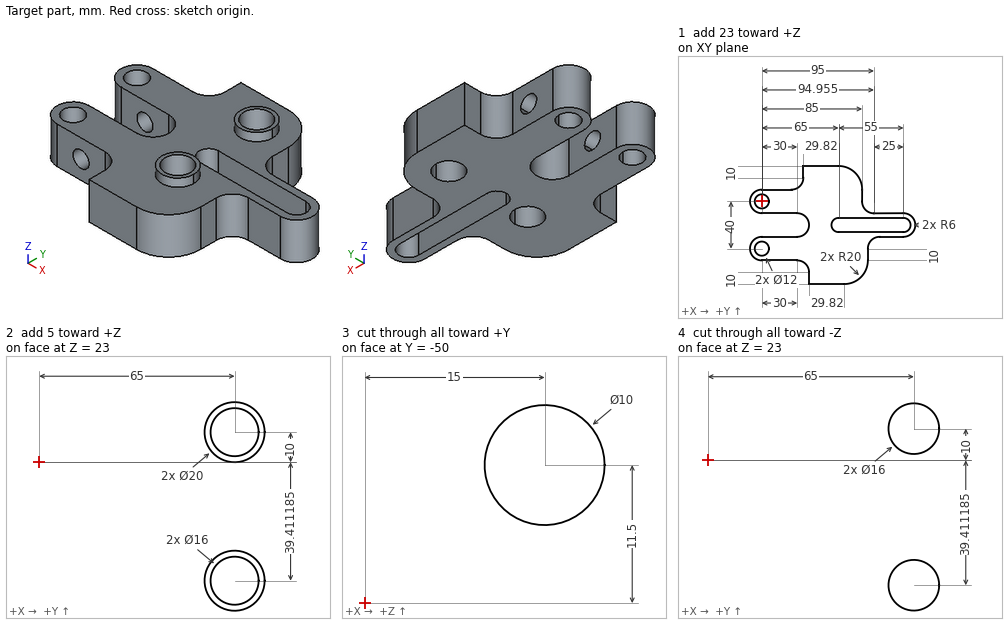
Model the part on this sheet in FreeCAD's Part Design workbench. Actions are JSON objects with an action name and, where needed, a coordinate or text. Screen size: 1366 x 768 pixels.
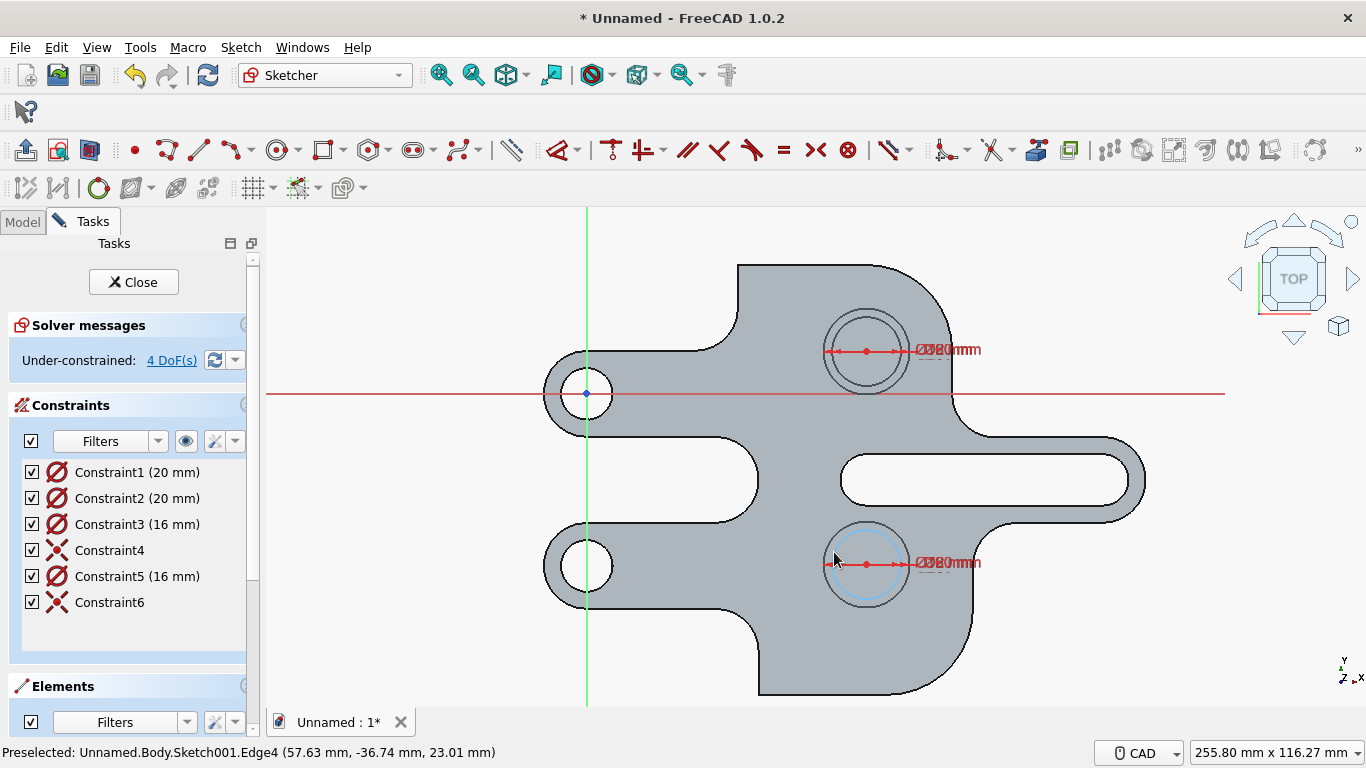
{"action": "left_click", "coordinate": [867, 352]}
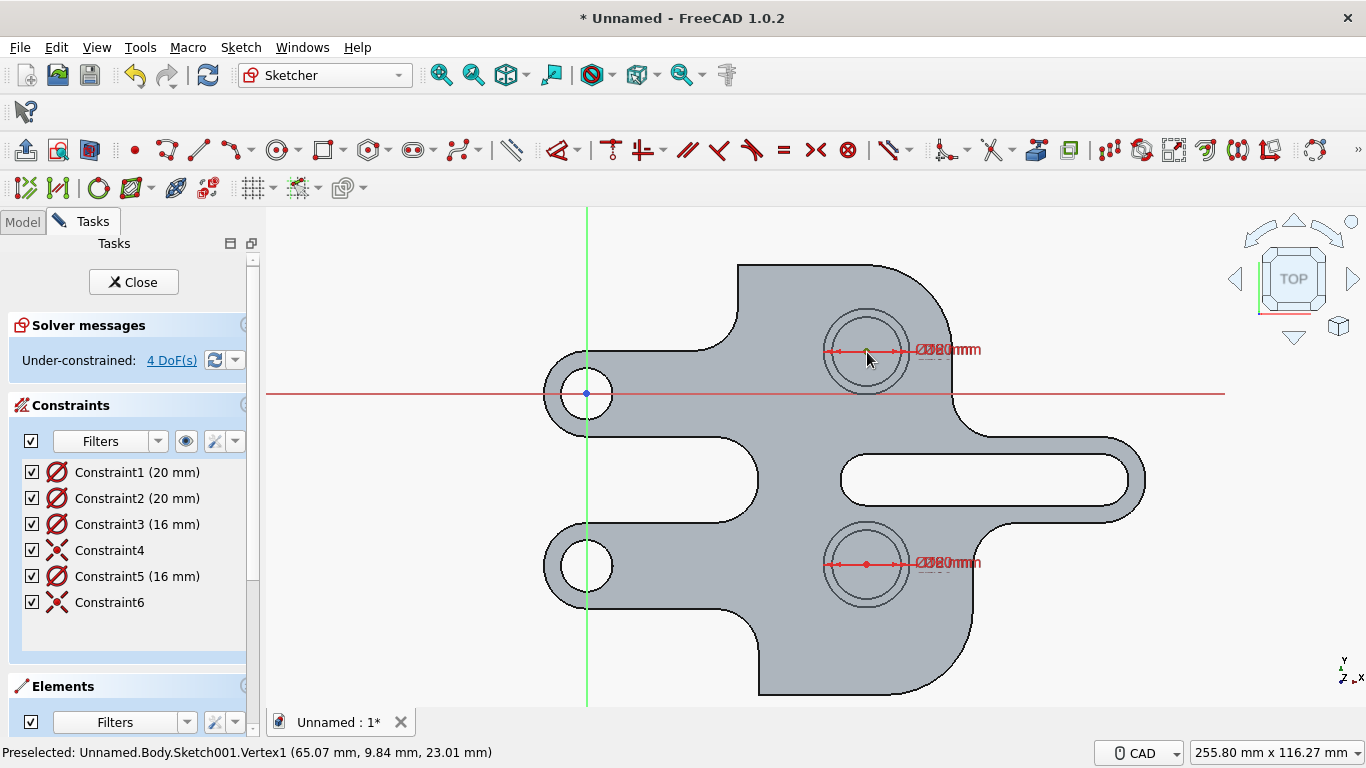
{"action": "left_click", "coordinate": [867, 565]}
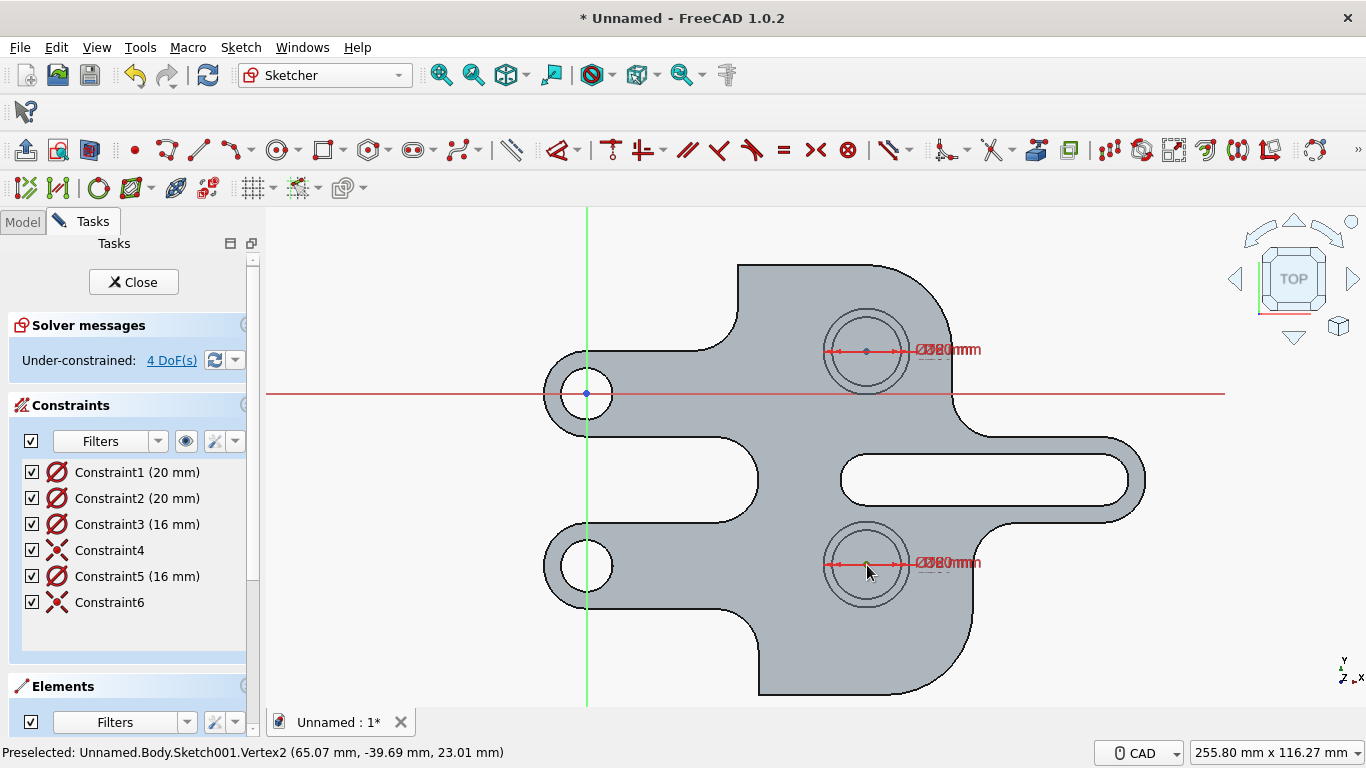
{"action": "key", "text": "v"}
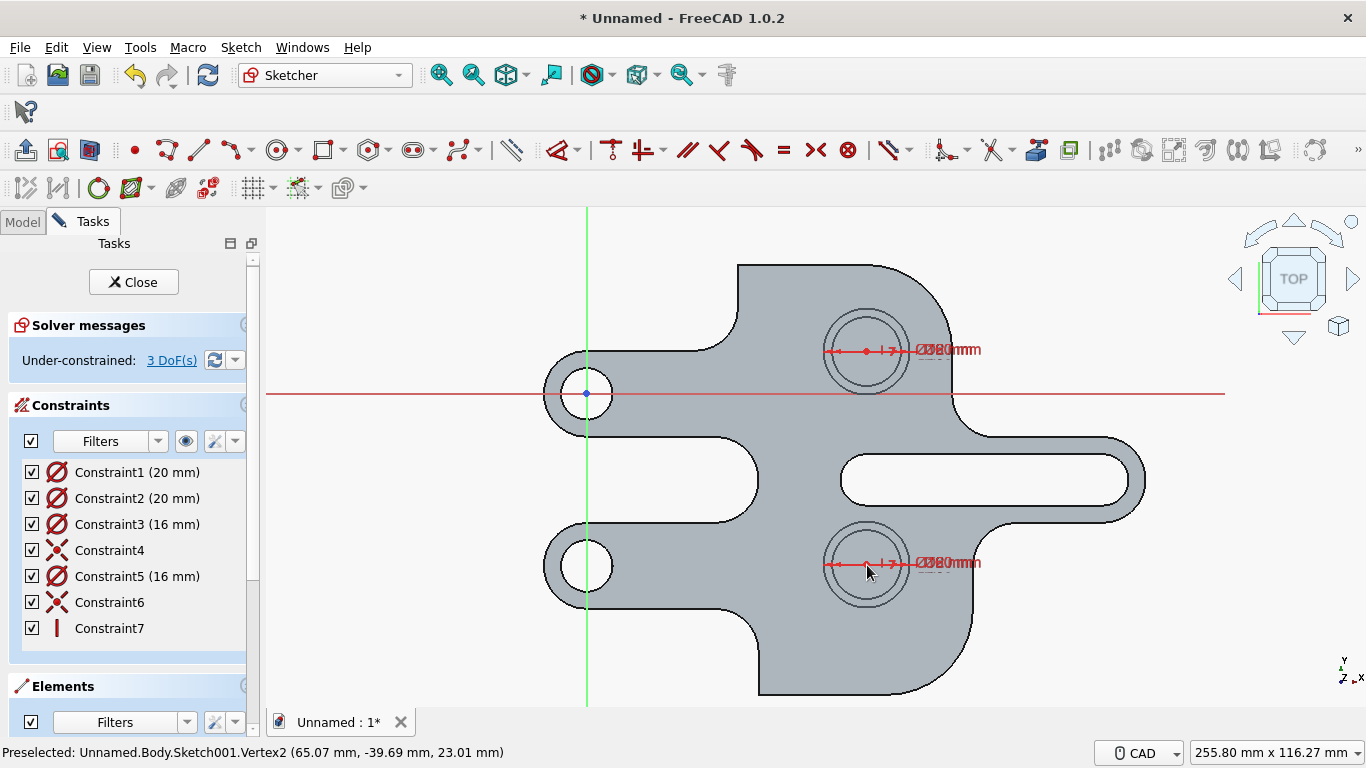
{"action": "left_click", "coordinate": [558, 150]}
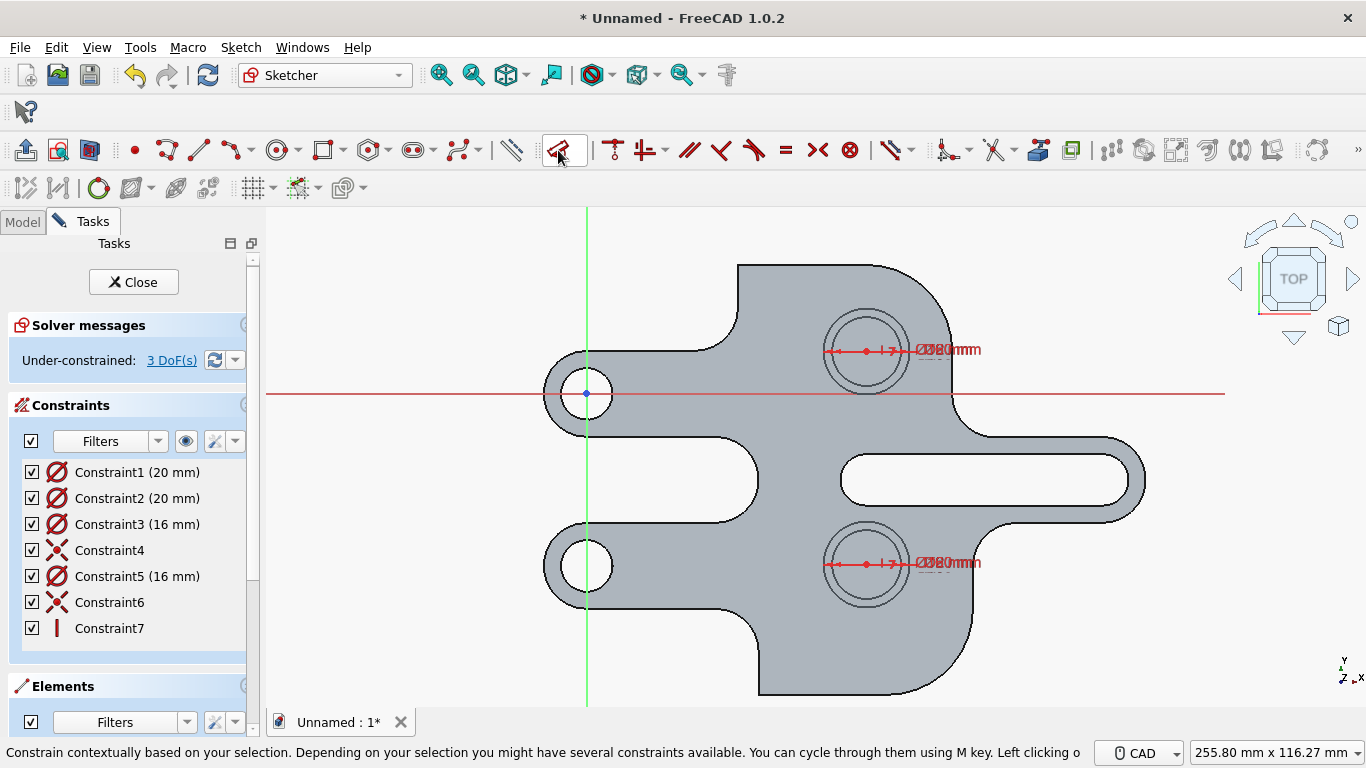
{"action": "left_click", "coordinate": [867, 352]}
{"action": "left_click", "coordinate": [727, 318]}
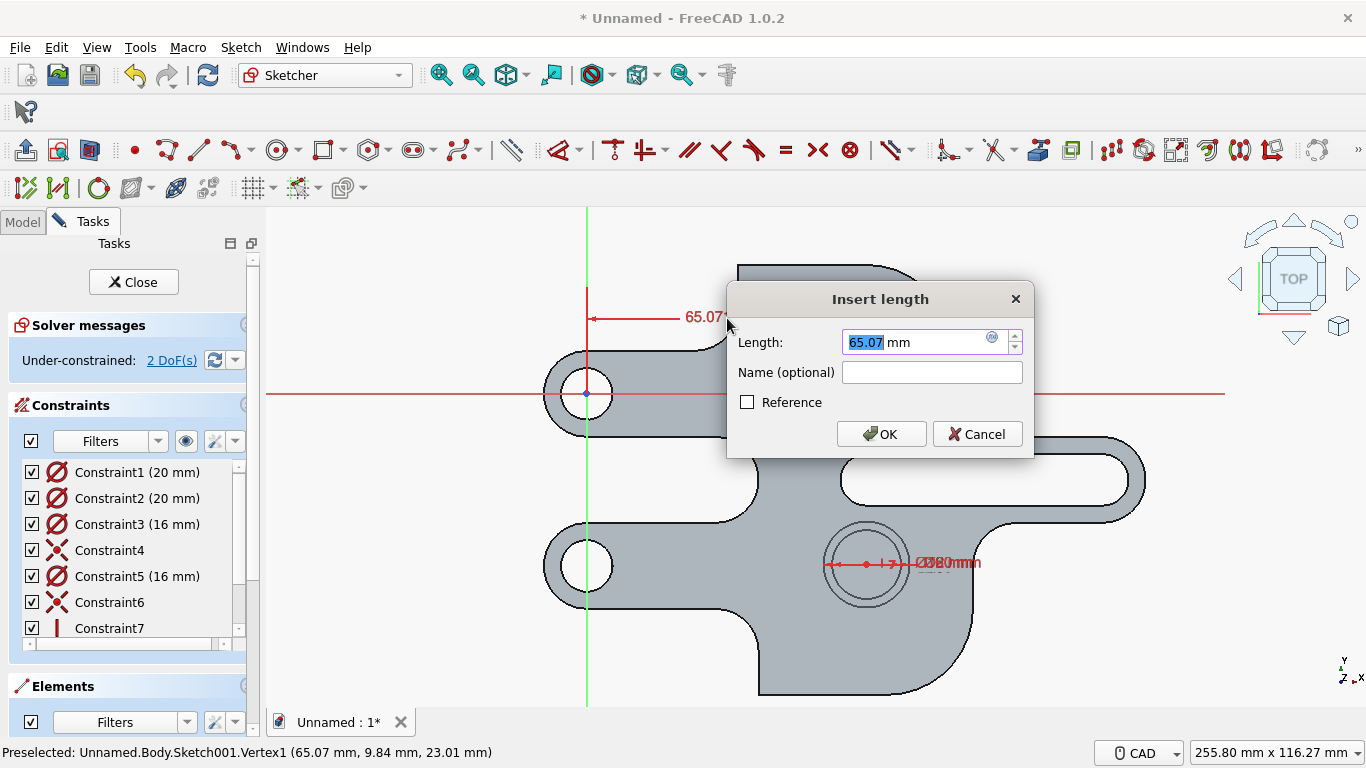
{"action": "type", "text": "65"}
{"action": "key", "text": "Return"}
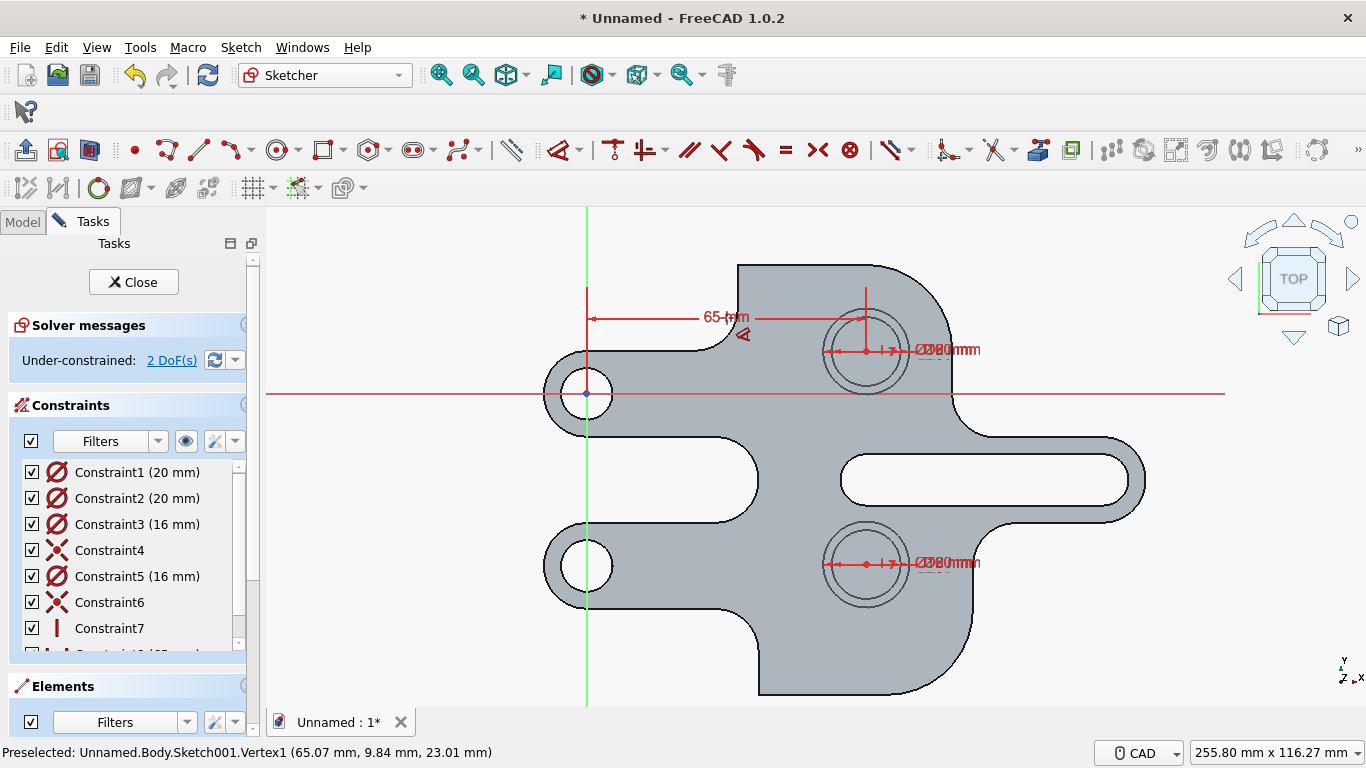
{"action": "left_click", "coordinate": [866, 352]}
{"action": "left_click", "coordinate": [553, 373]}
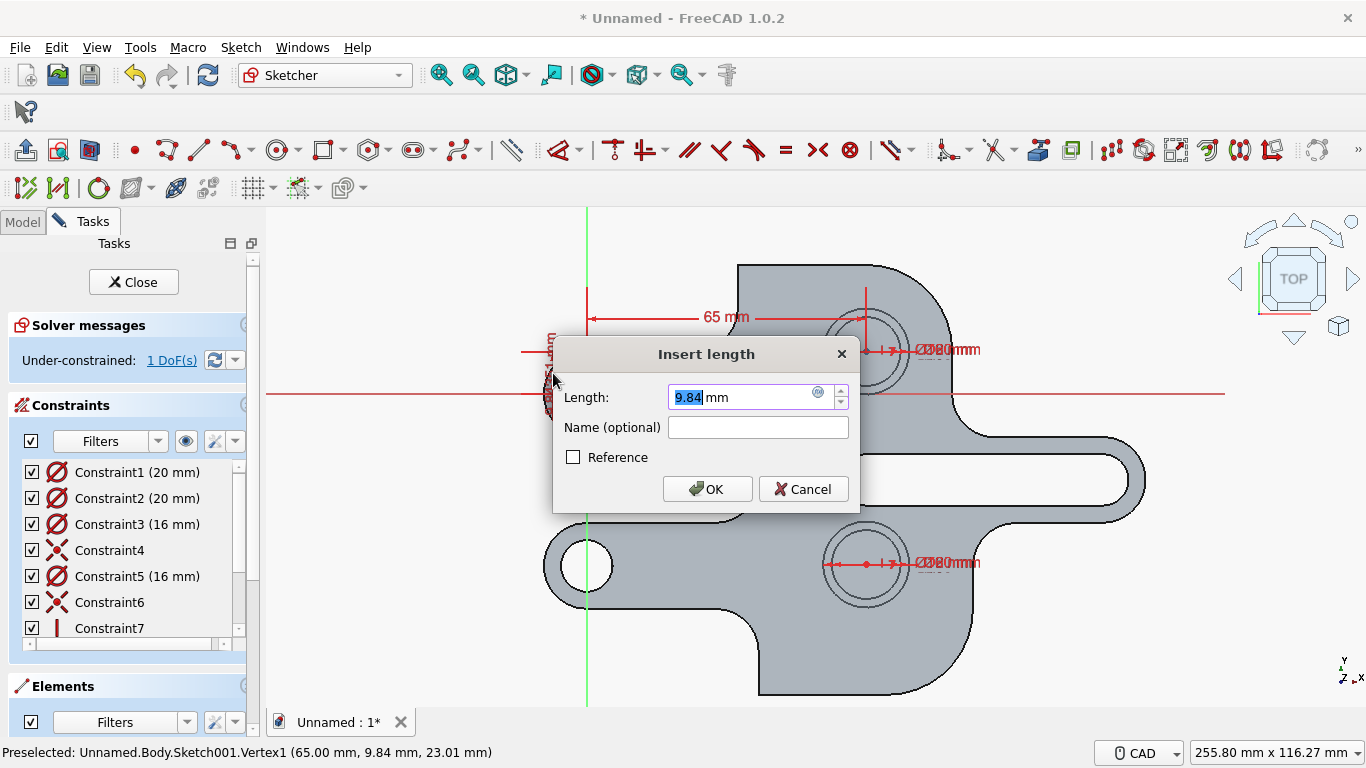
{"action": "type", "text": "10"}
{"action": "key", "text": "Return"}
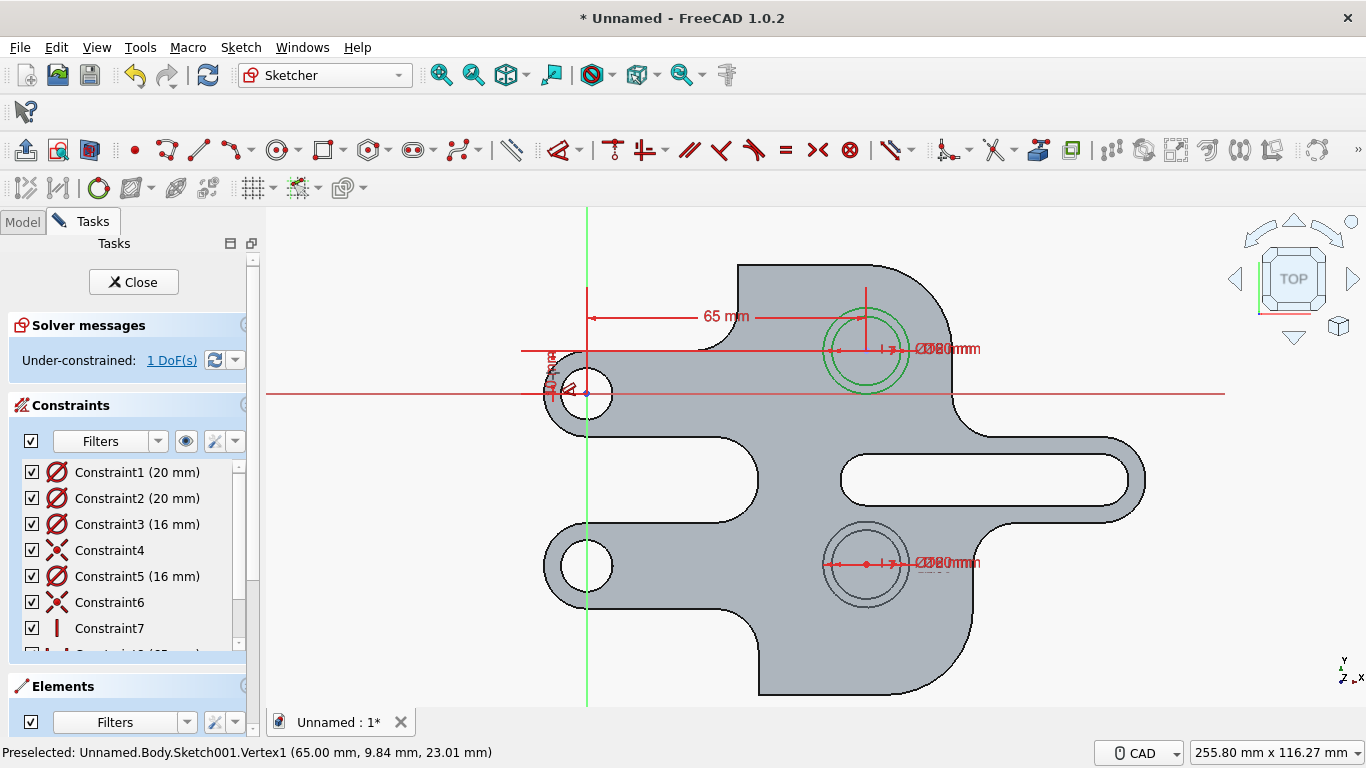
{"action": "left_click", "coordinate": [866, 565]}
{"action": "left_click", "coordinate": [553, 479]}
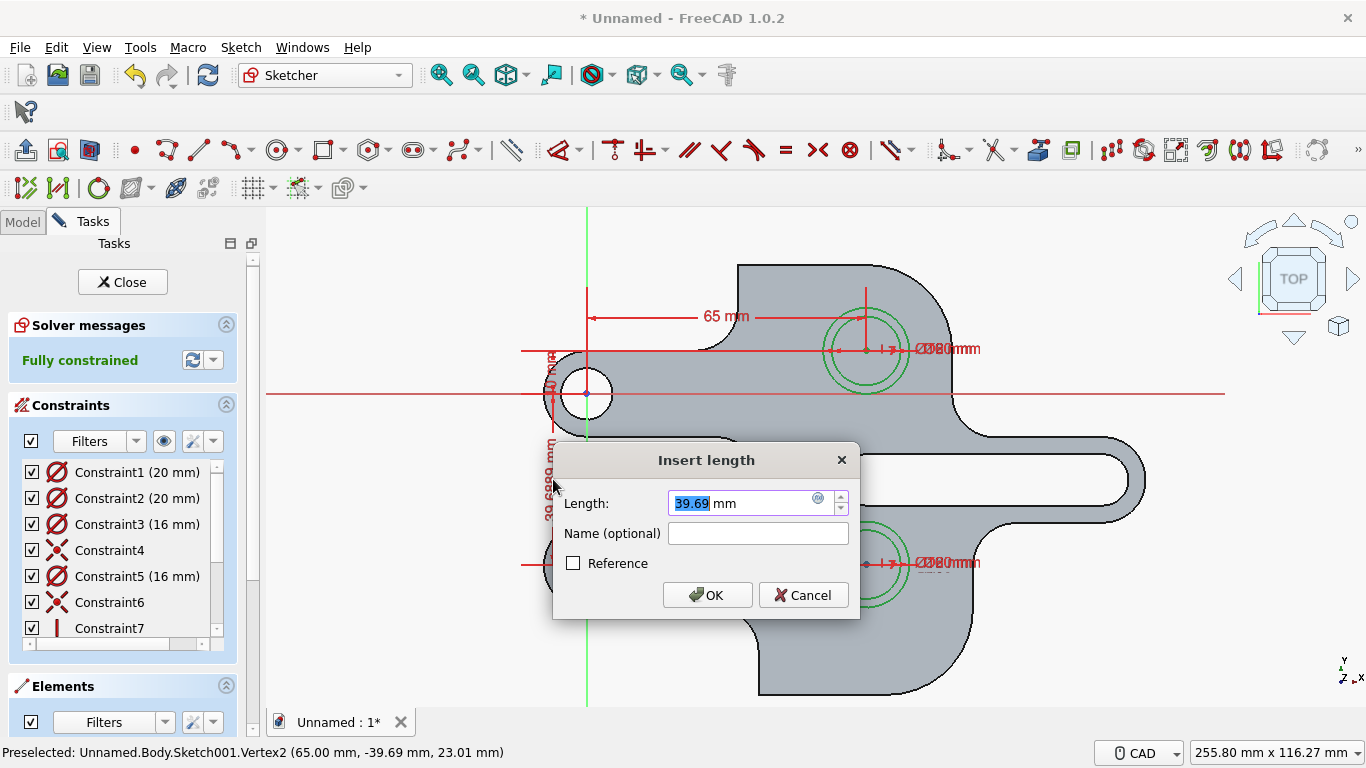
{"action": "type", "text": "39.411185"}
{"action": "key", "text": "Return"}
{"action": "key", "text": "Escape"}